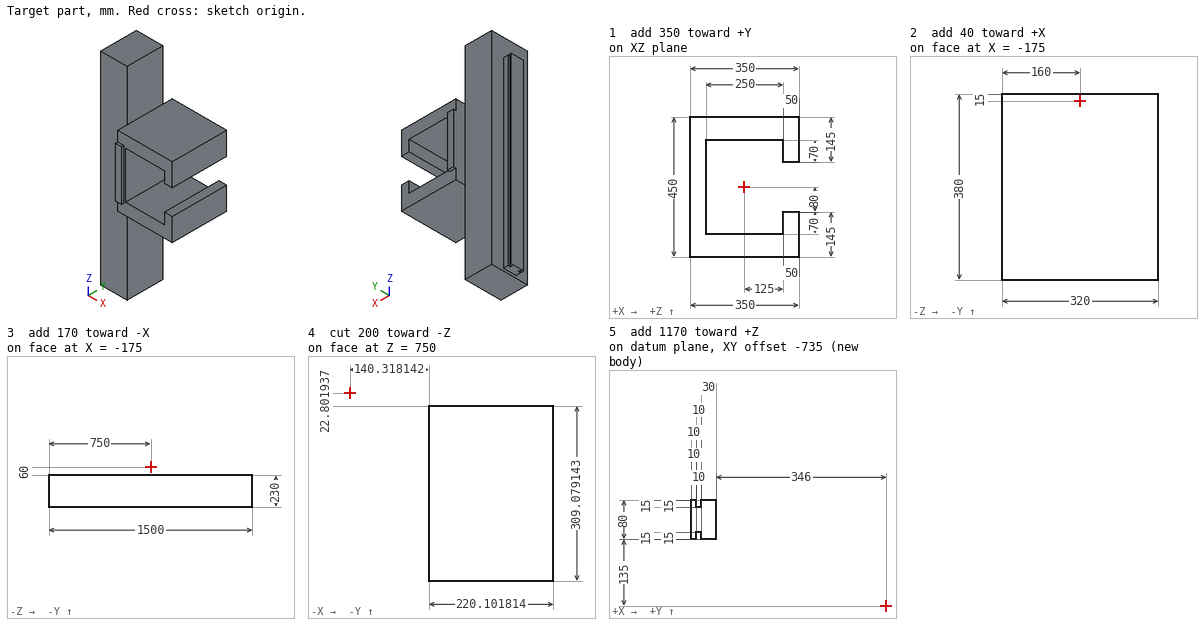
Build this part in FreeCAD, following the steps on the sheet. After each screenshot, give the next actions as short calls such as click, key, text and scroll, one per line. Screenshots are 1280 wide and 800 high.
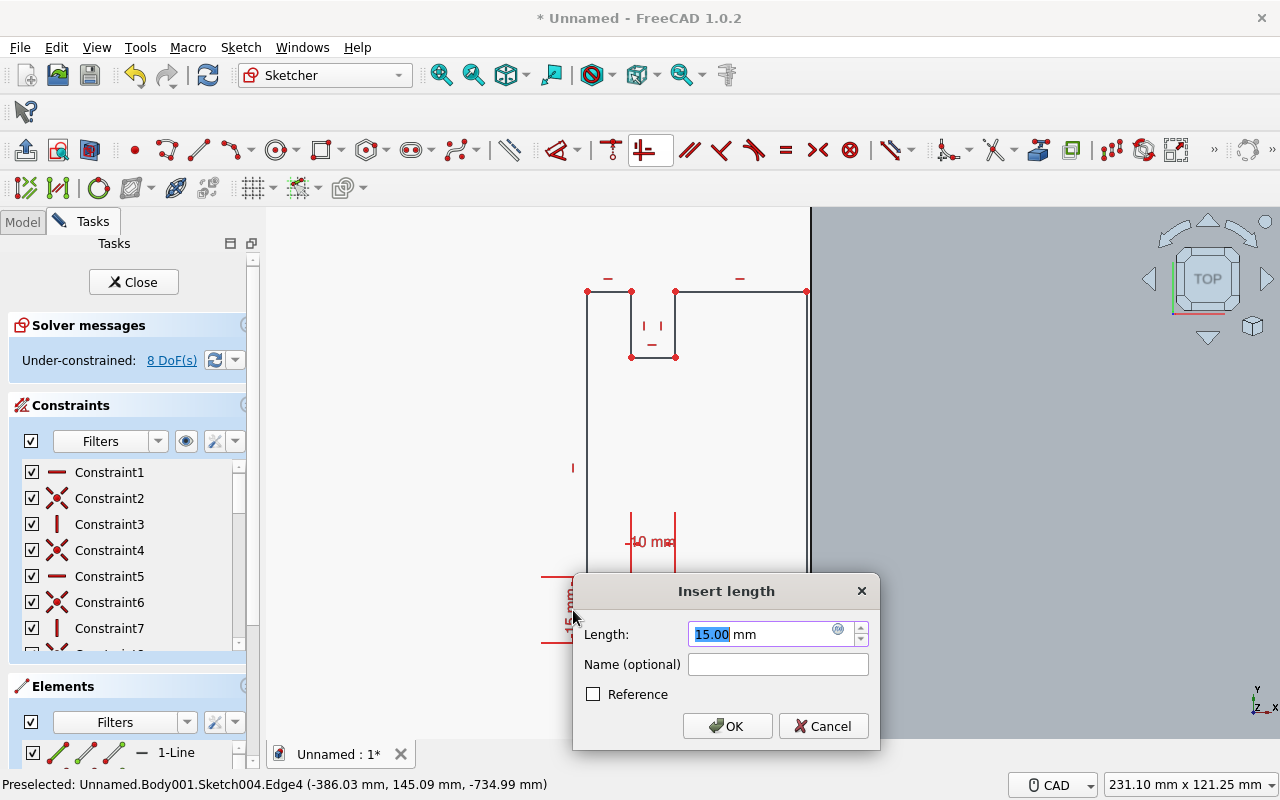
text(15)
key(Return)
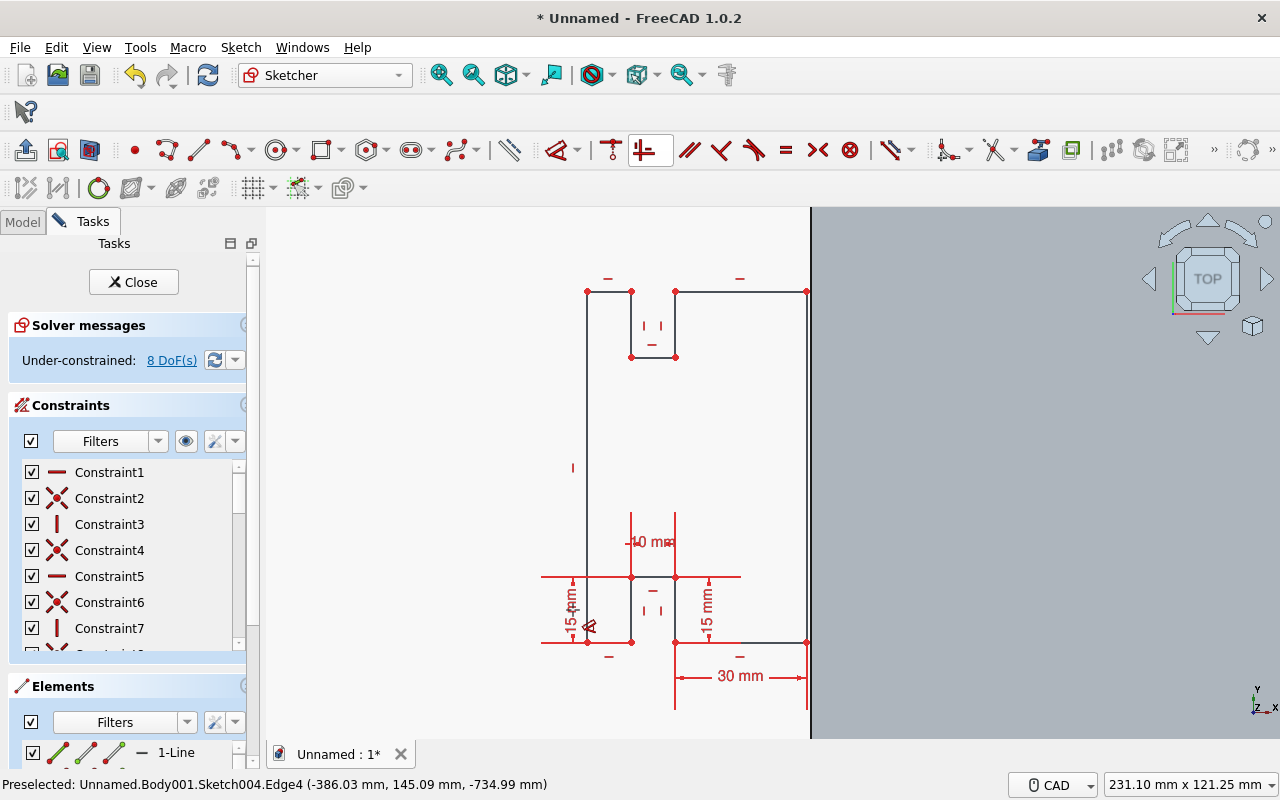
click(618, 643)
click(609, 677)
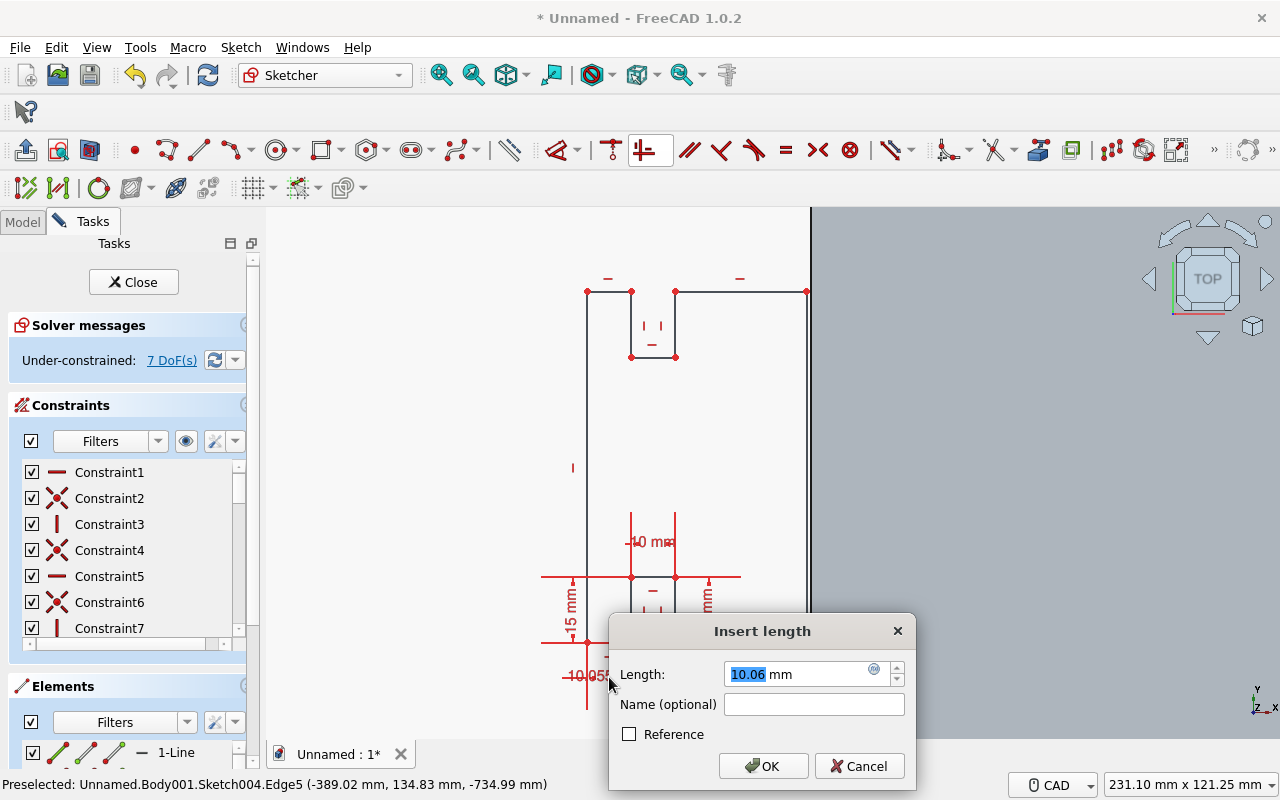
text(10)
key(Return)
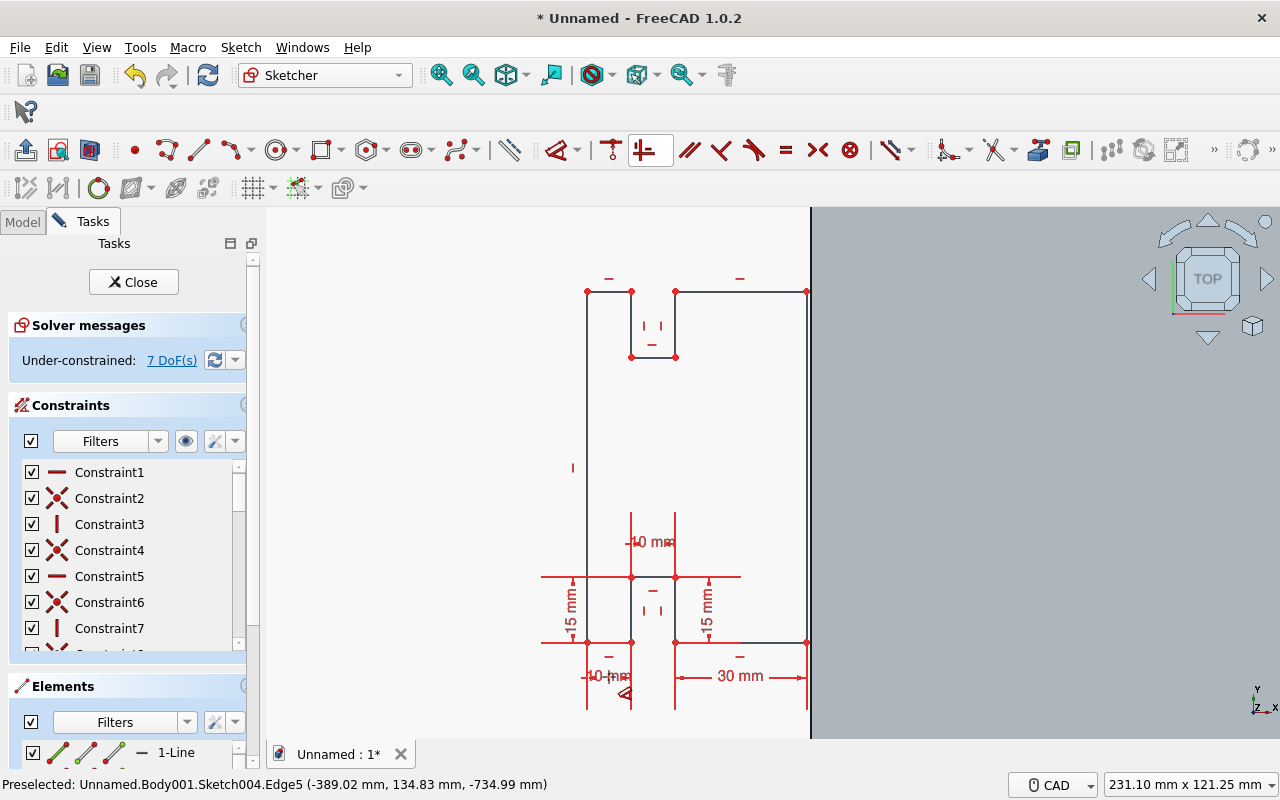
click(587, 538)
click(553, 468)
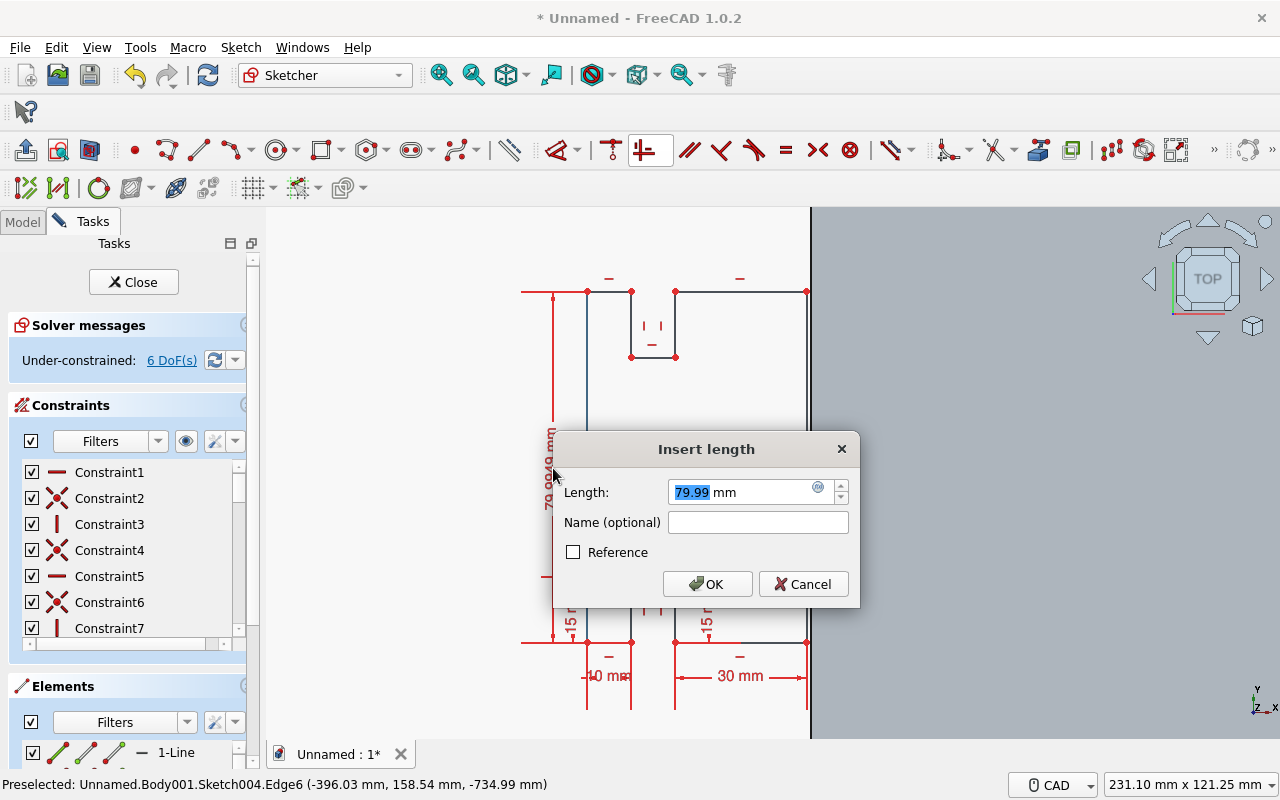
text(80)
key(Return)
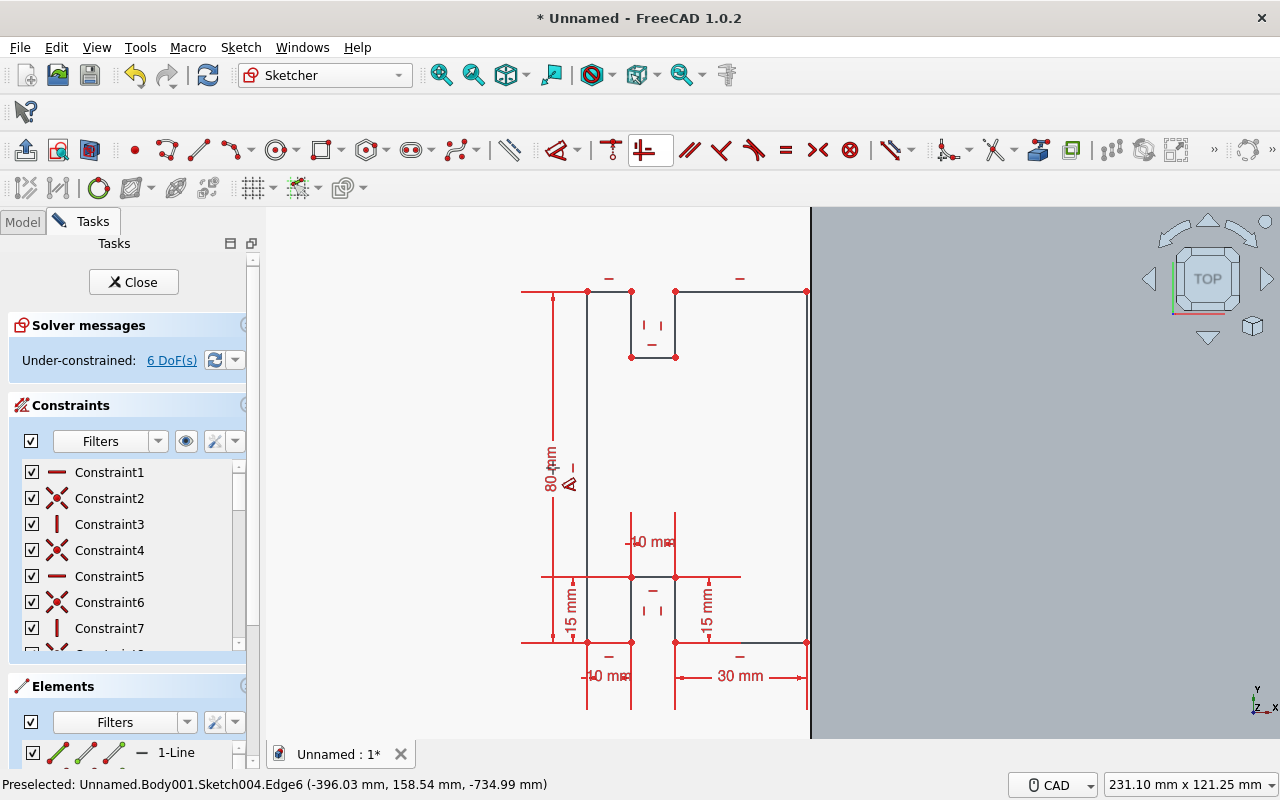
click(600, 292)
click(609, 258)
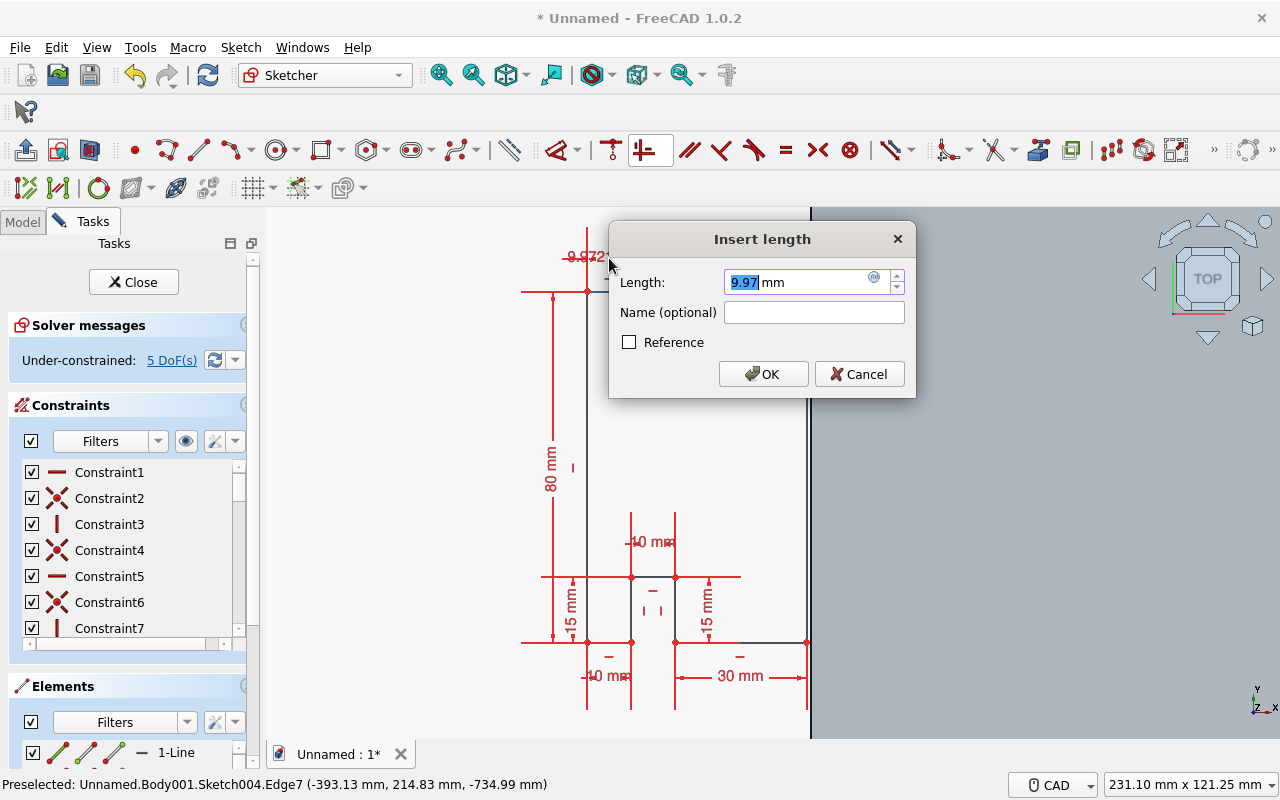
text(10)
key(Return)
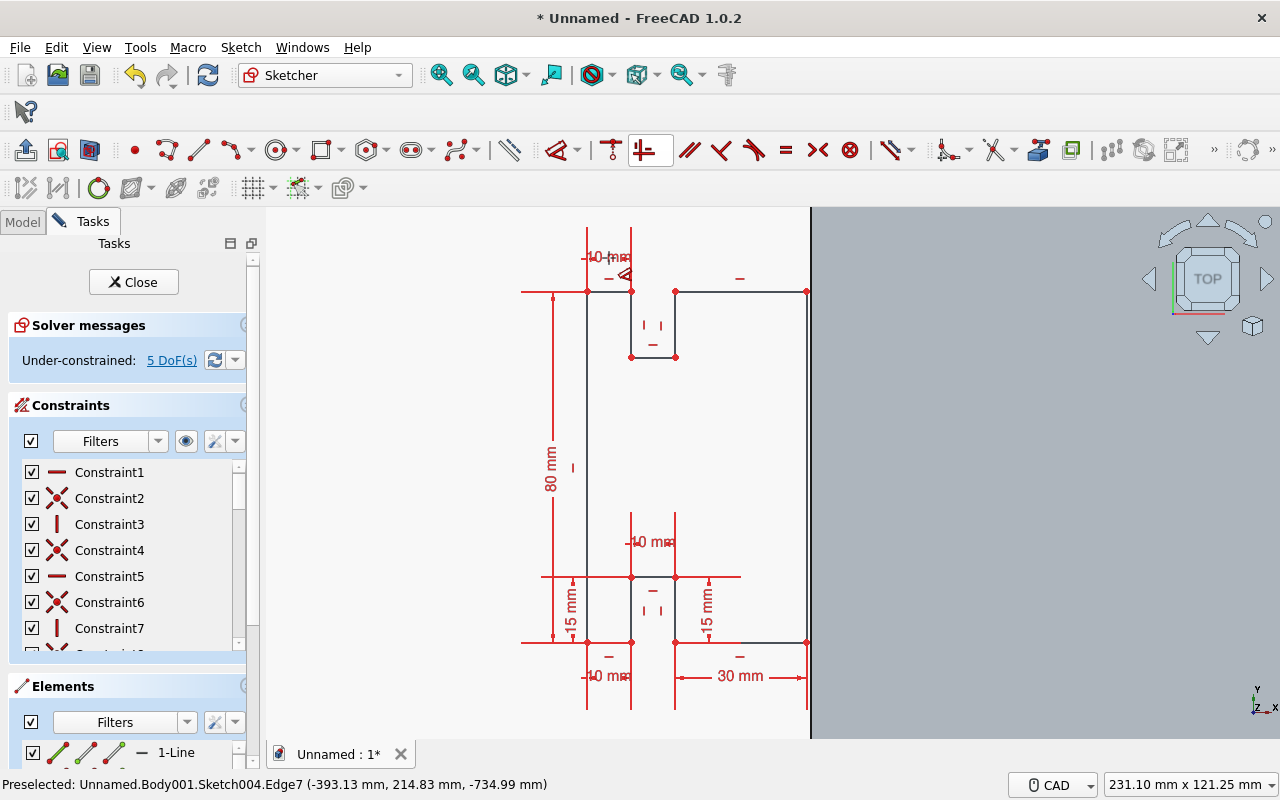
click(631, 312)
click(573, 325)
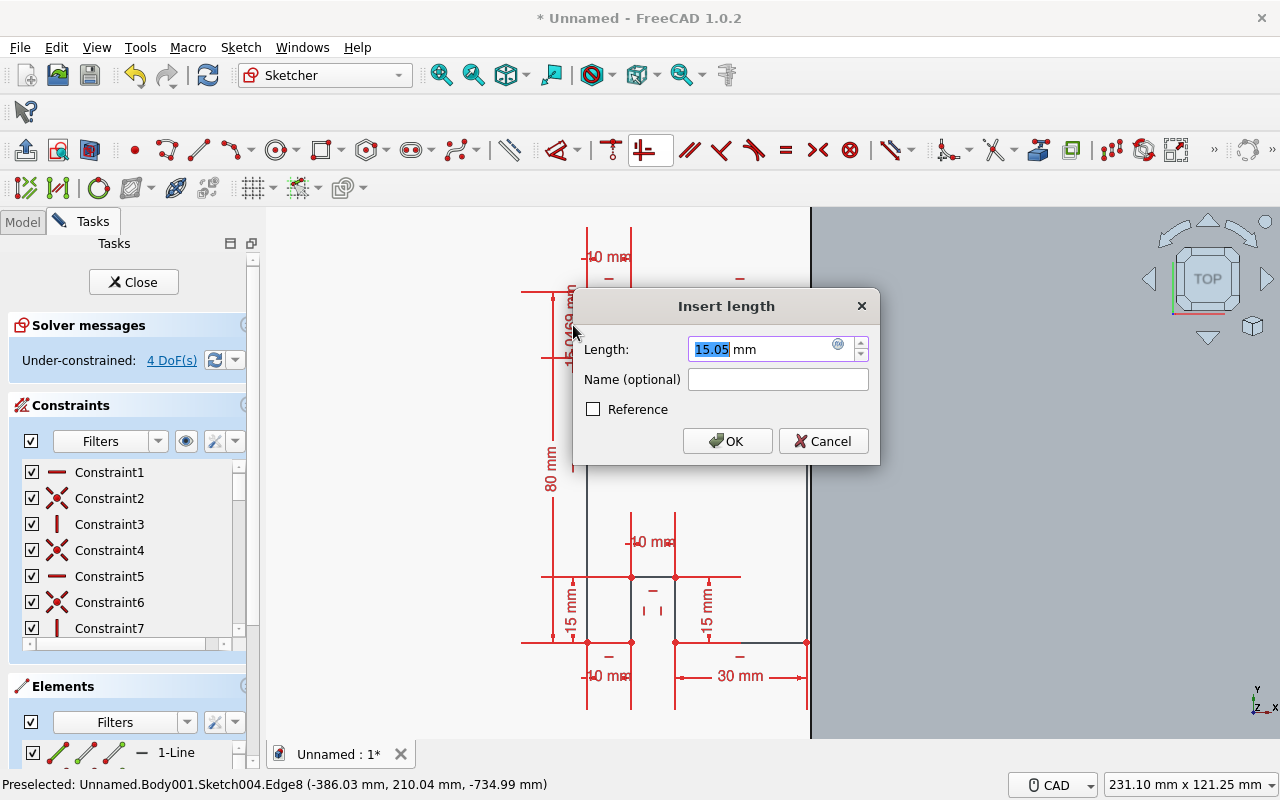
text(15)
key(Return)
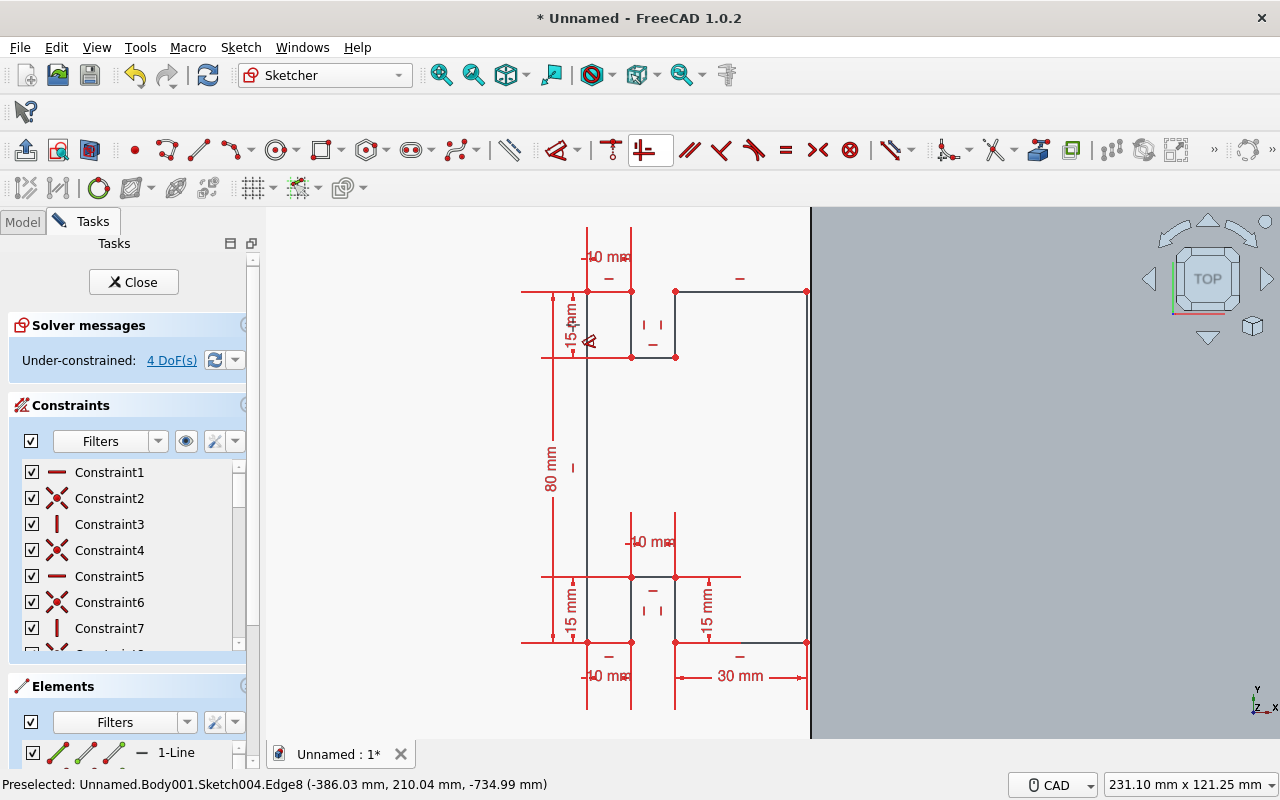
click(644, 358)
click(653, 324)